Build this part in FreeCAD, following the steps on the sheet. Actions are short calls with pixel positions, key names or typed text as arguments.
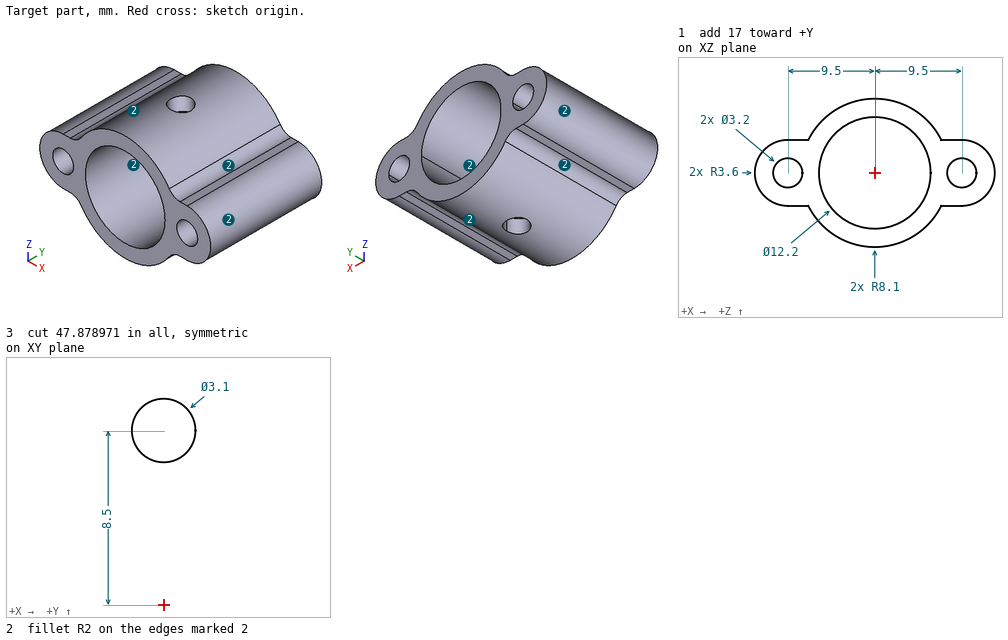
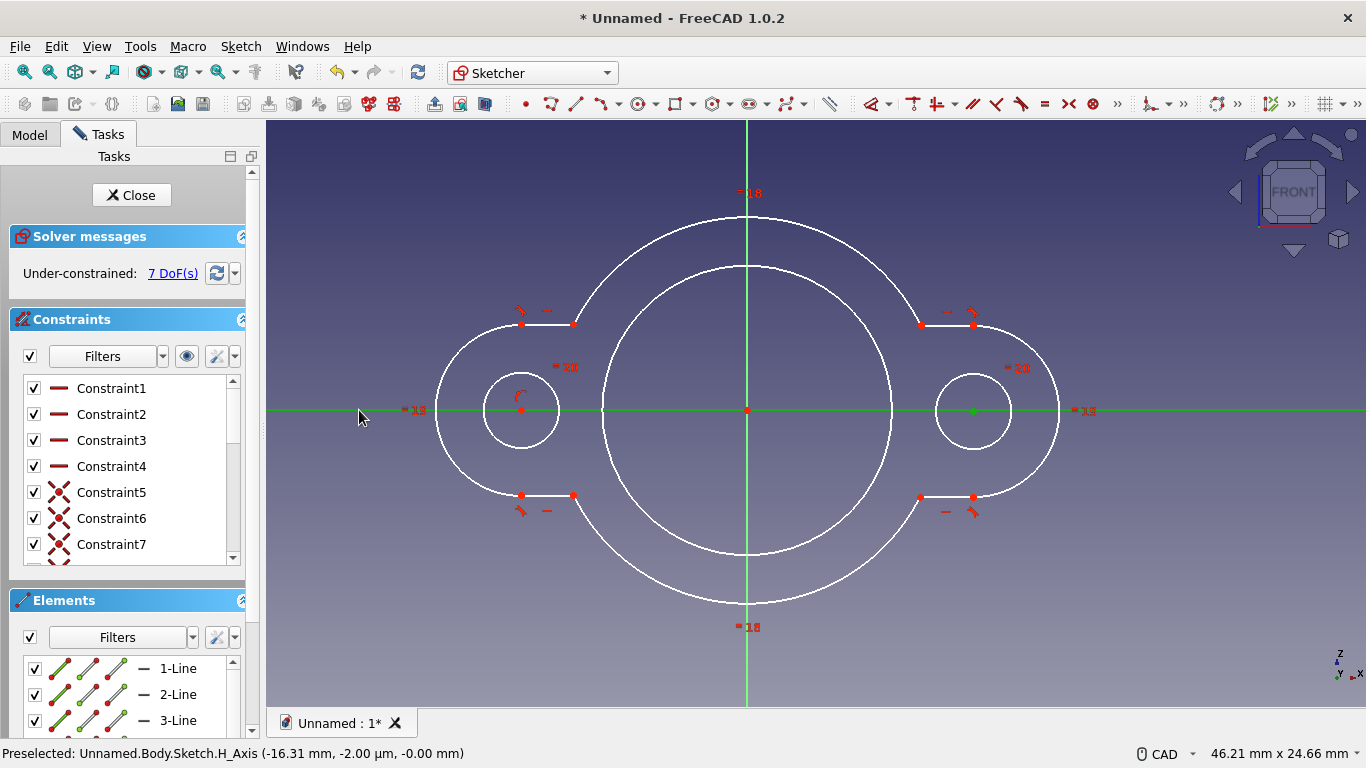
key(c)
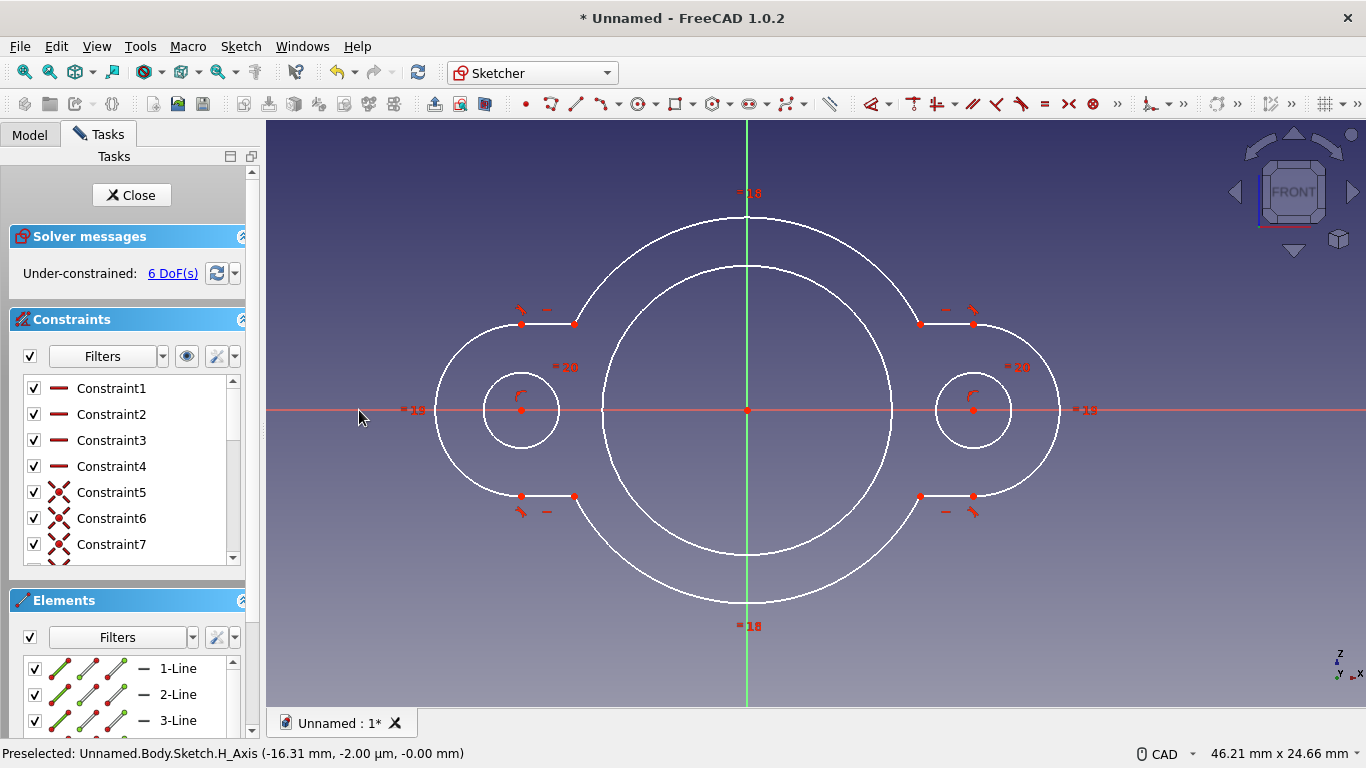
click(664, 585)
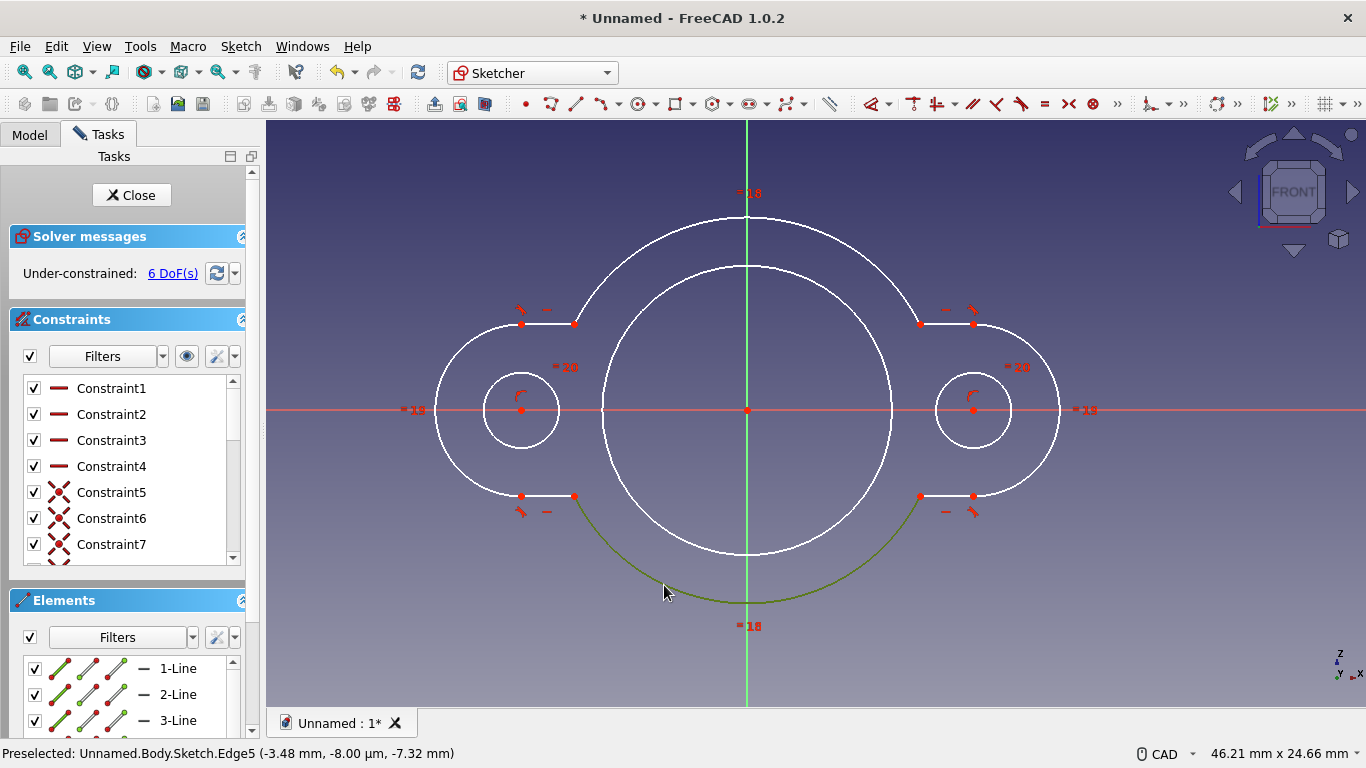
key(k)
key(r)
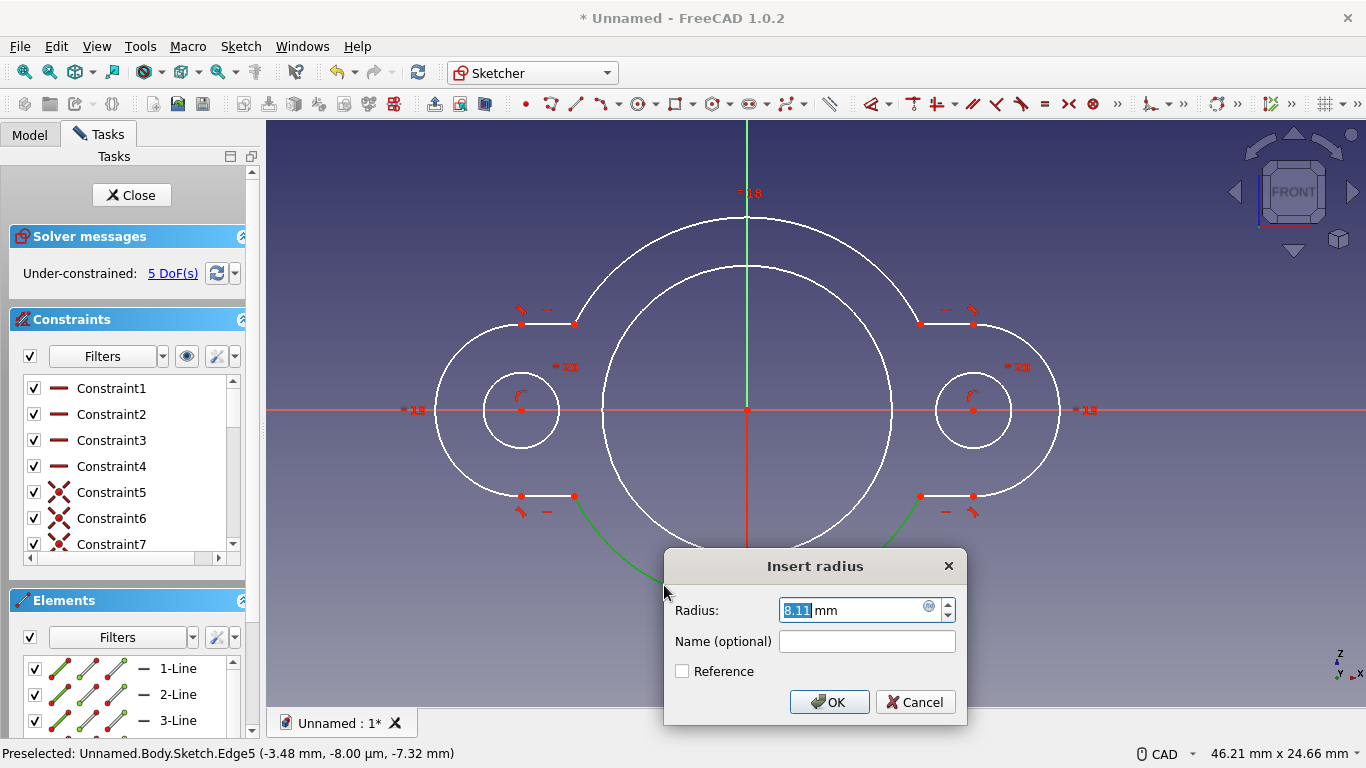
text(8.1)
key(Return)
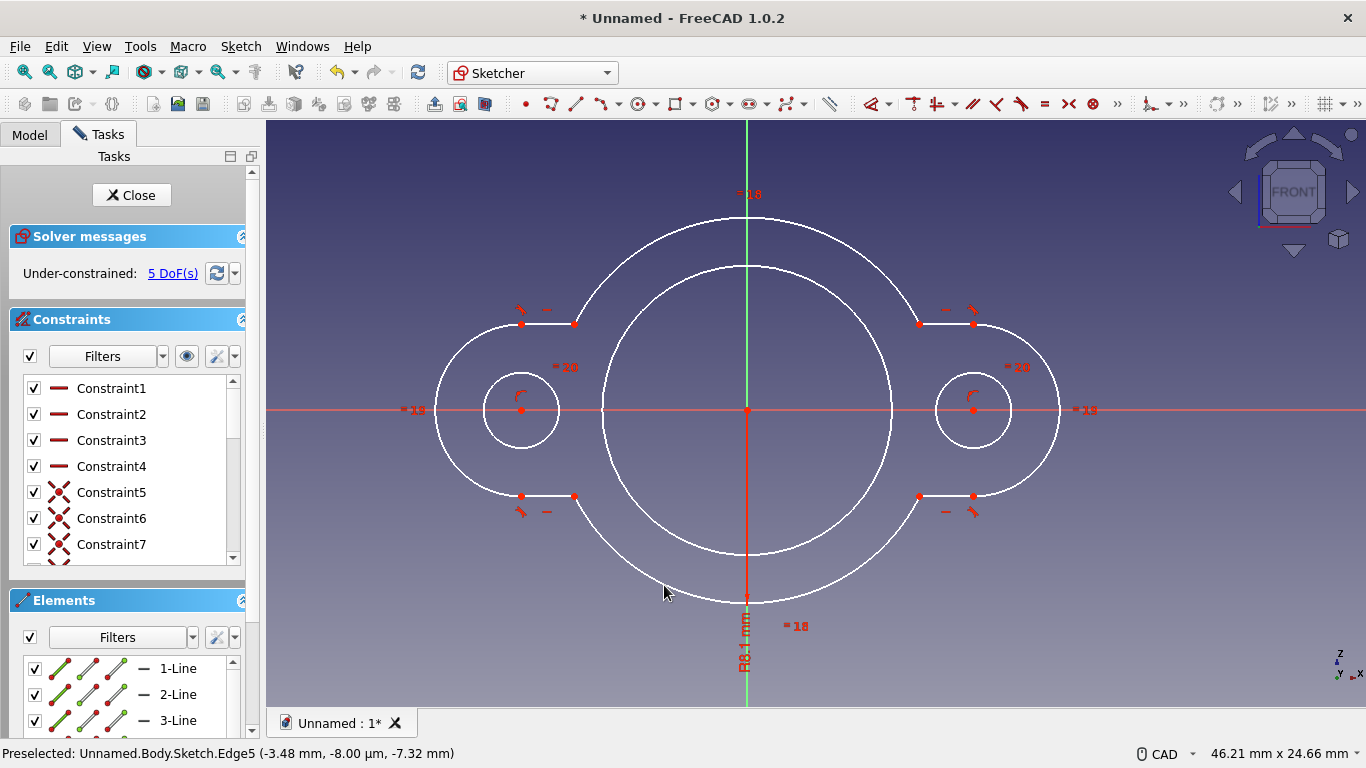
click(452, 360)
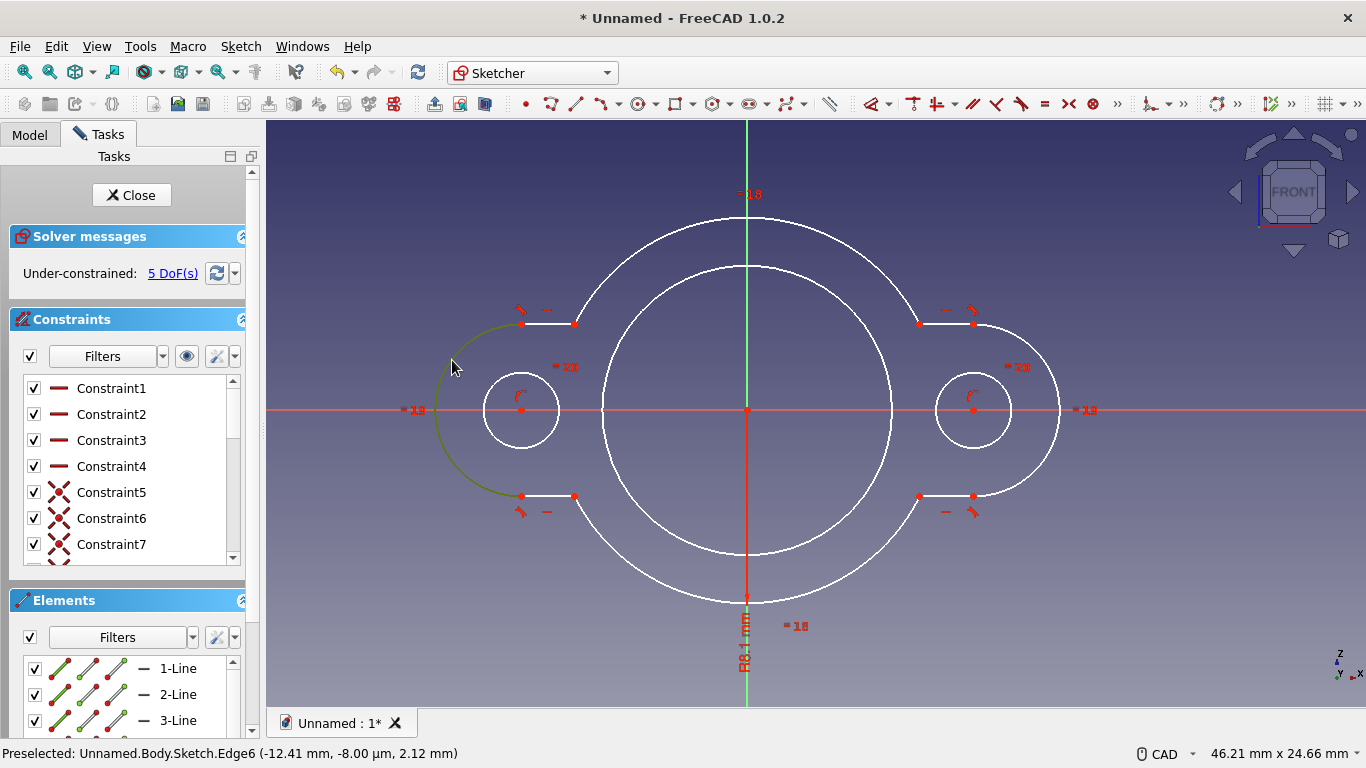
key(k)
key(r)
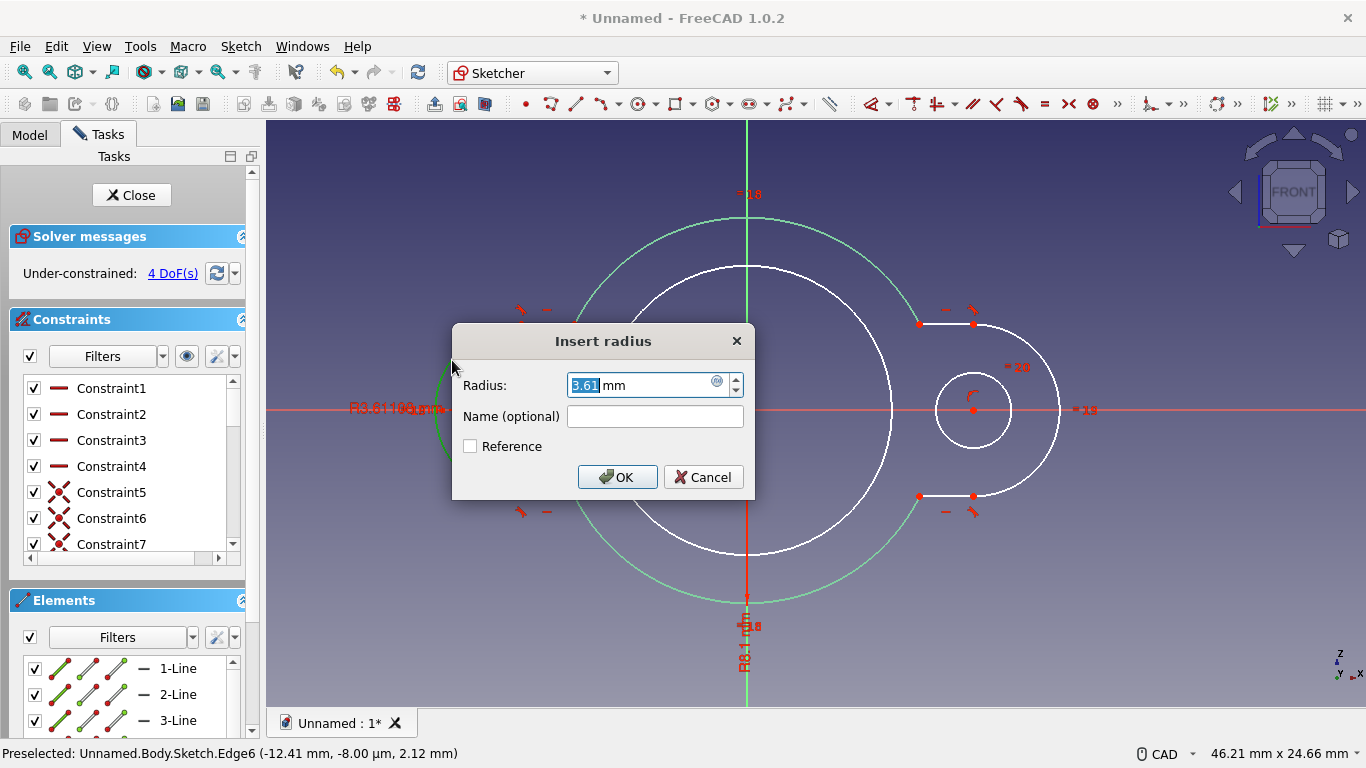
text(3.6)
key(Return)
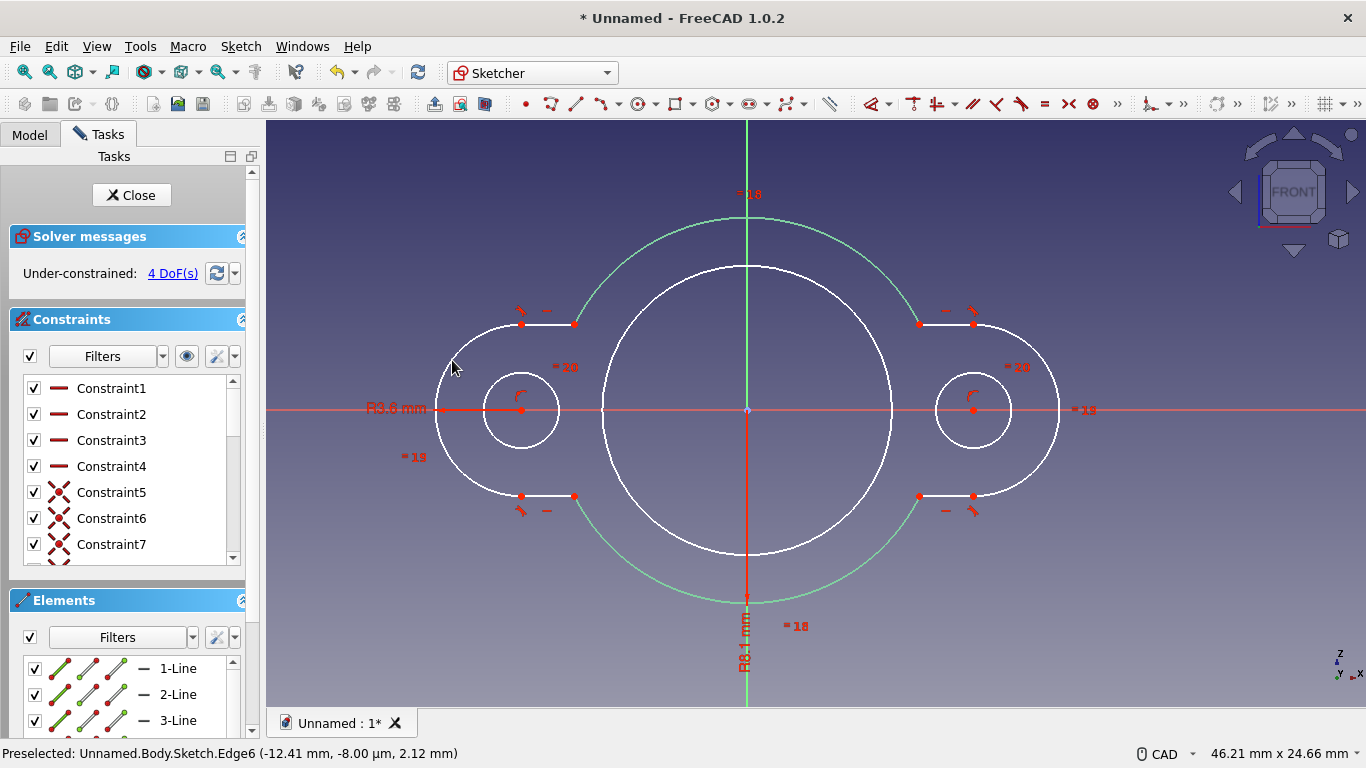
click(548, 384)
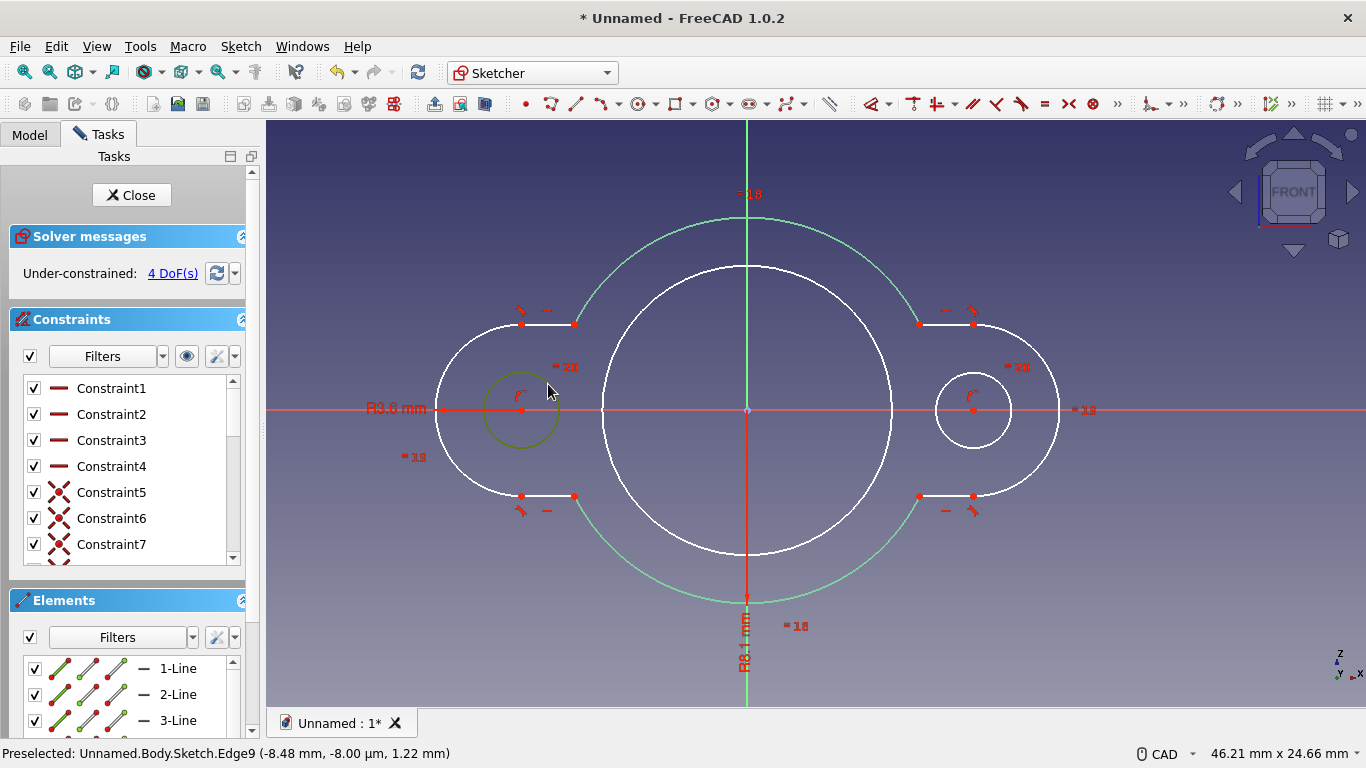
key(k)
key(o)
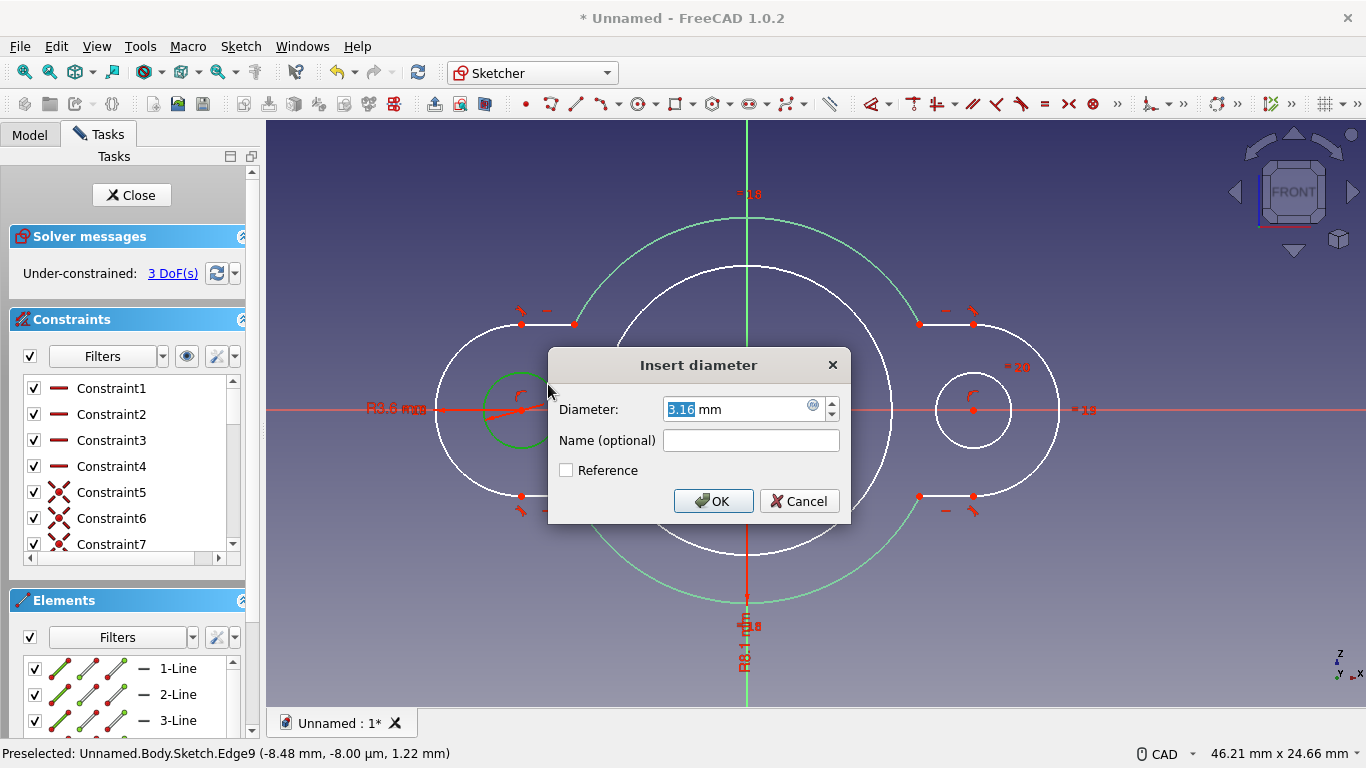
text(3.2)
key(Return)